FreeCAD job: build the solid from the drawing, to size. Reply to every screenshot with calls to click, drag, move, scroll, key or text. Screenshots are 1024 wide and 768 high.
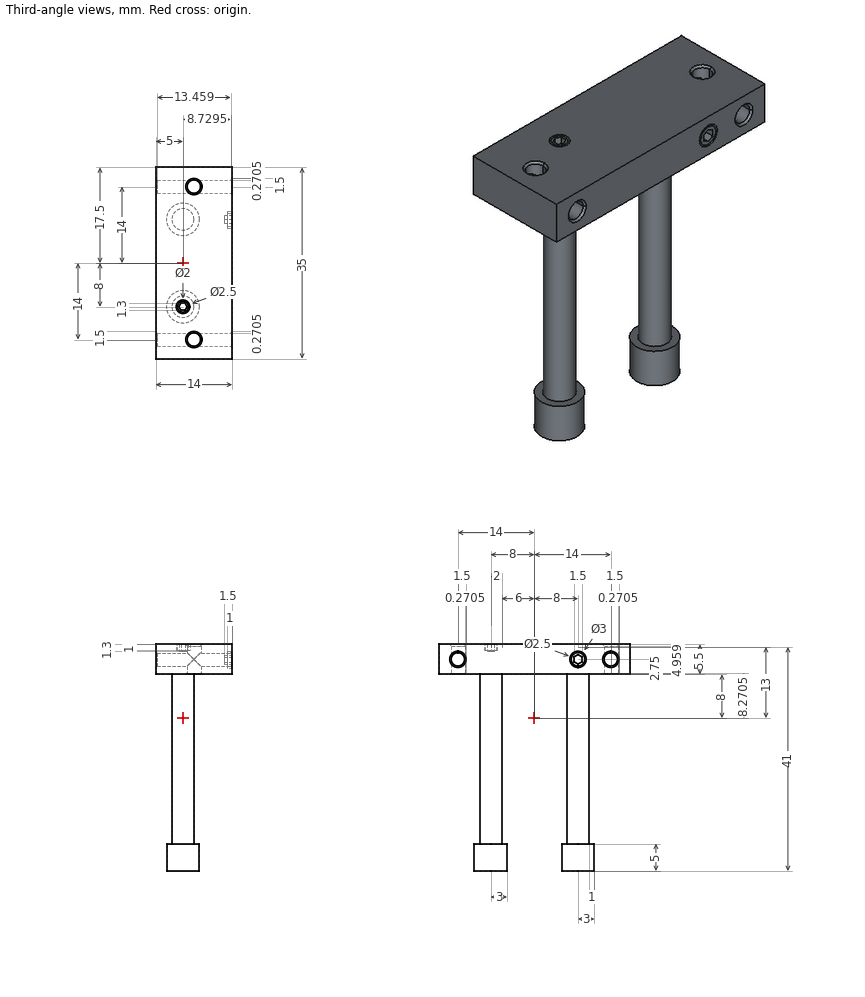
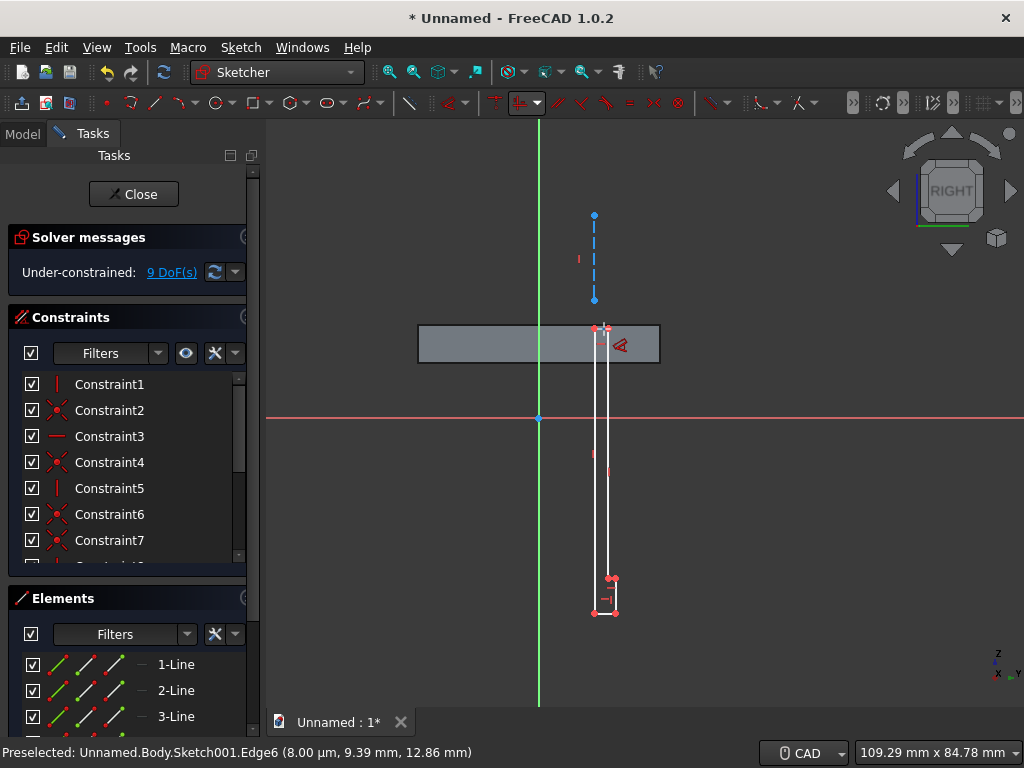
scroll(601, 614, up, 4)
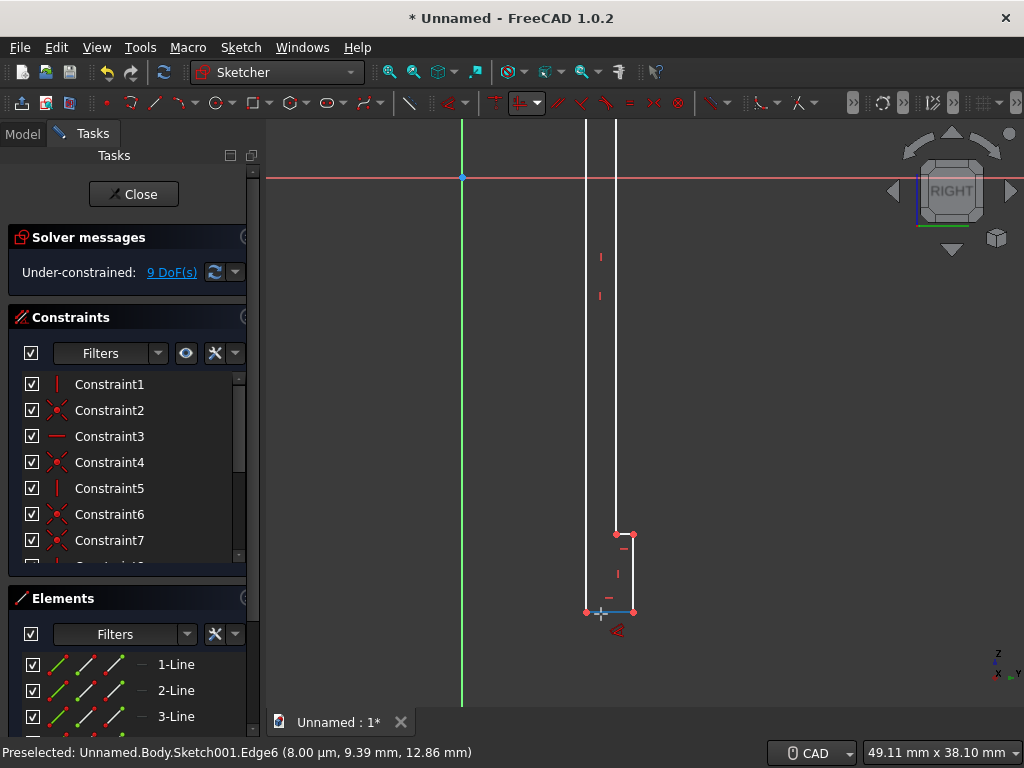
click(600, 612)
click(610, 646)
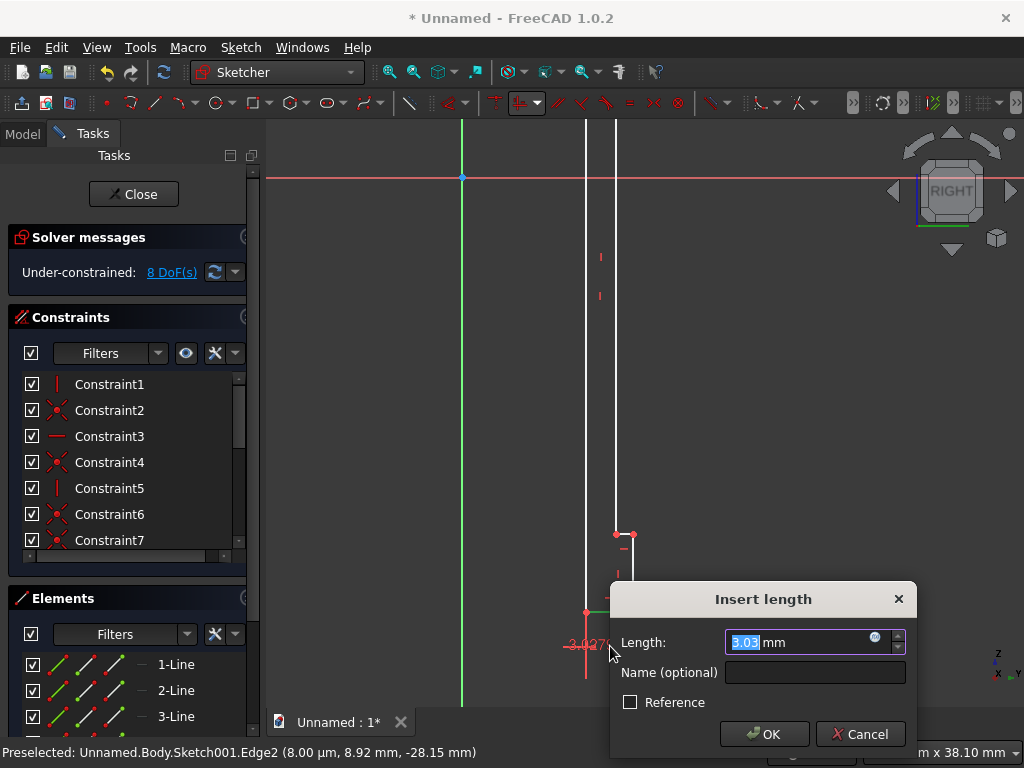
text(3)
key(Return)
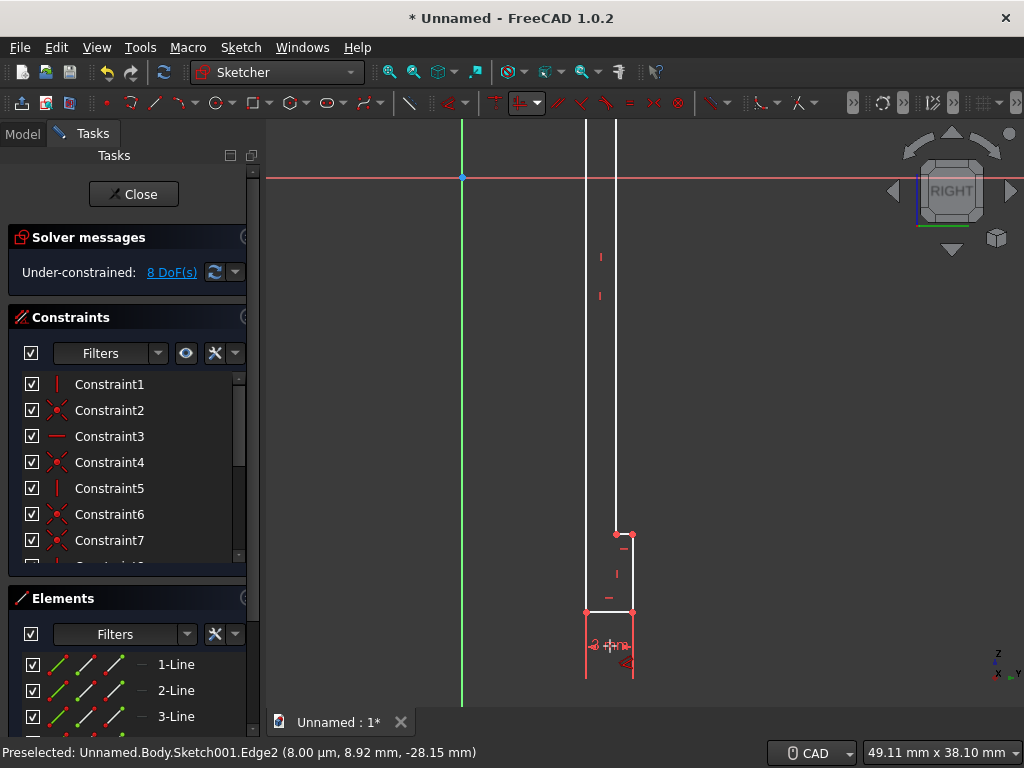
click(633, 589)
click(667, 573)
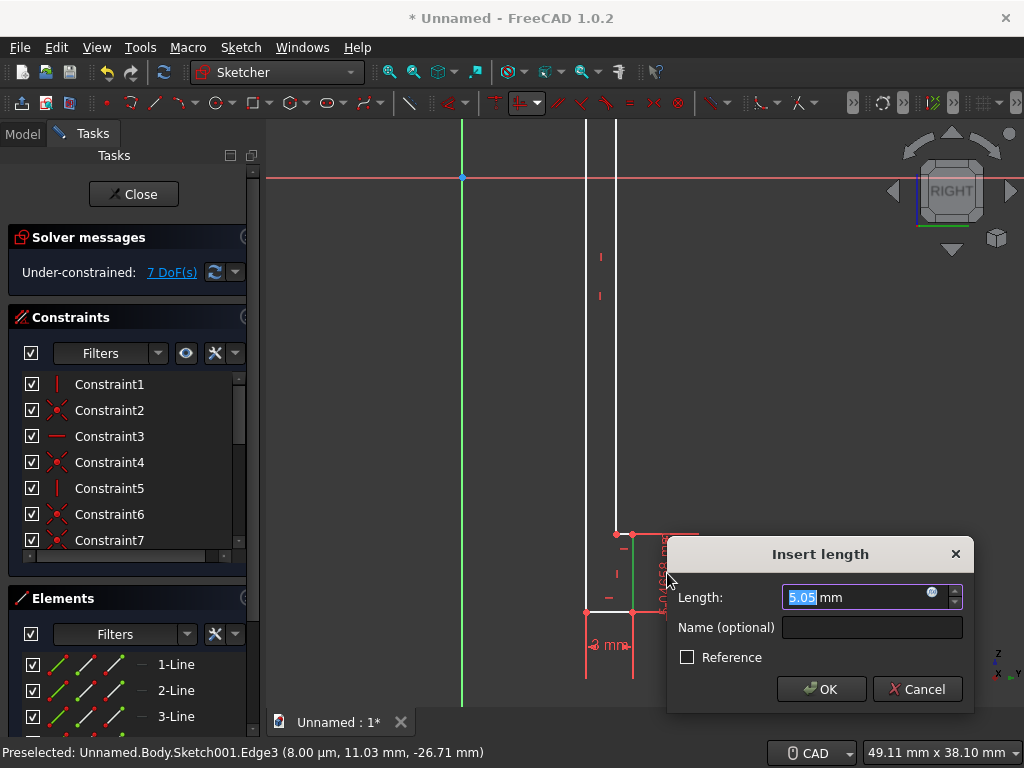
text(5)
key(Return)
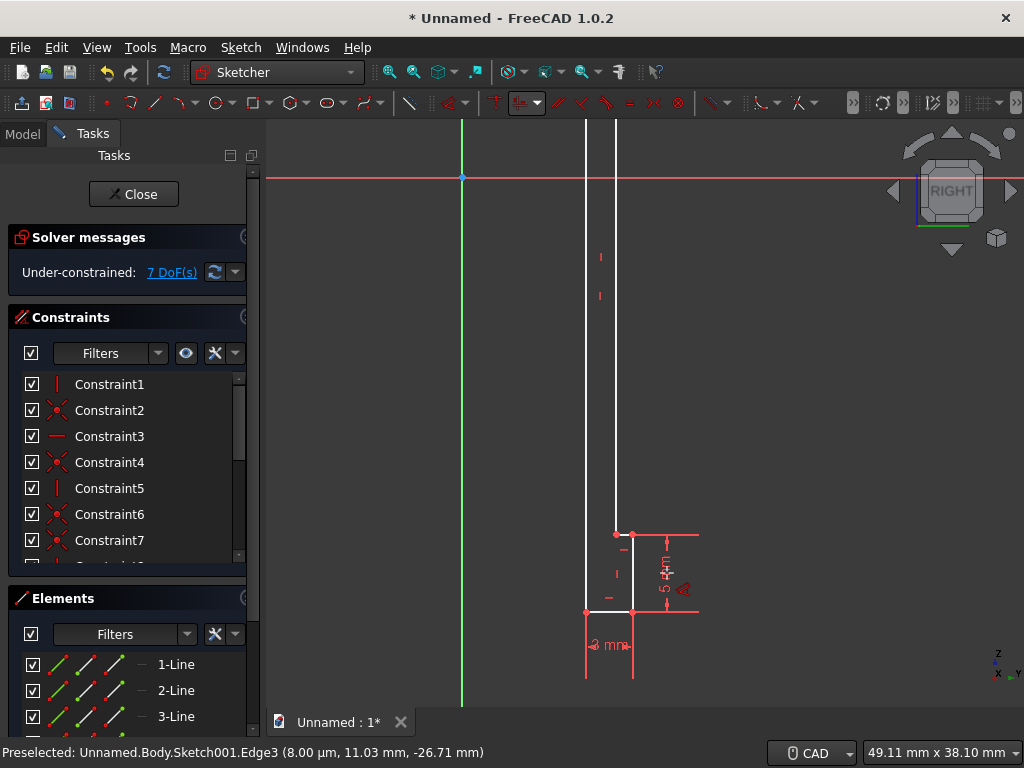
scroll(625, 535, up, 5)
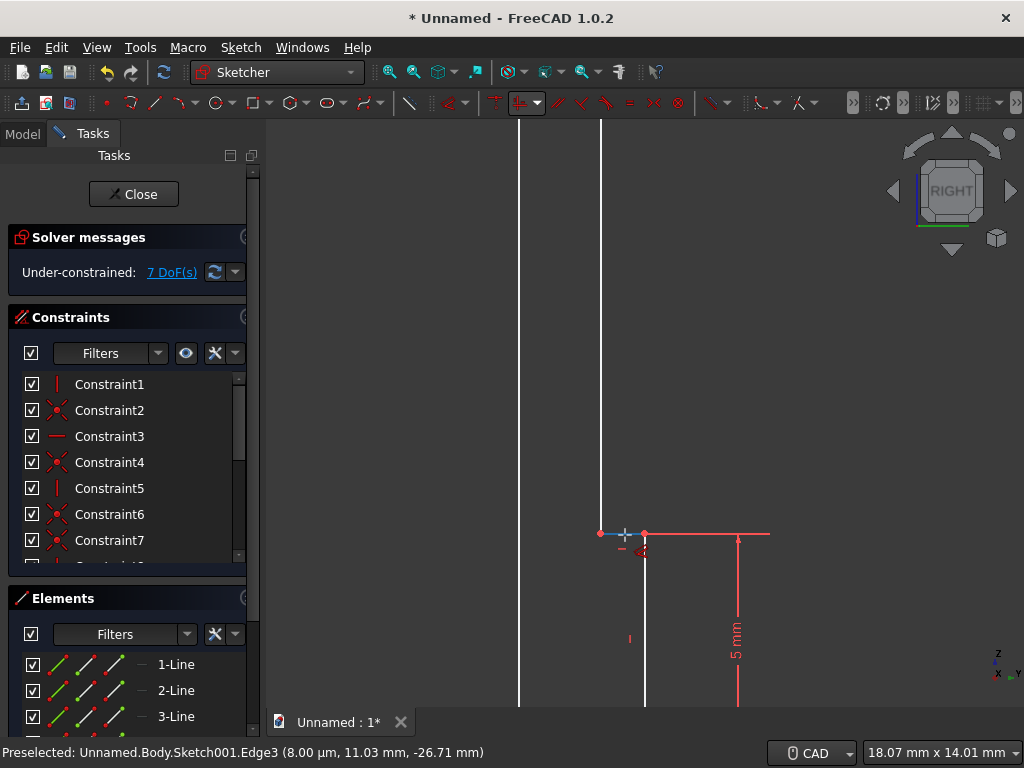
click(623, 534)
click(623, 568)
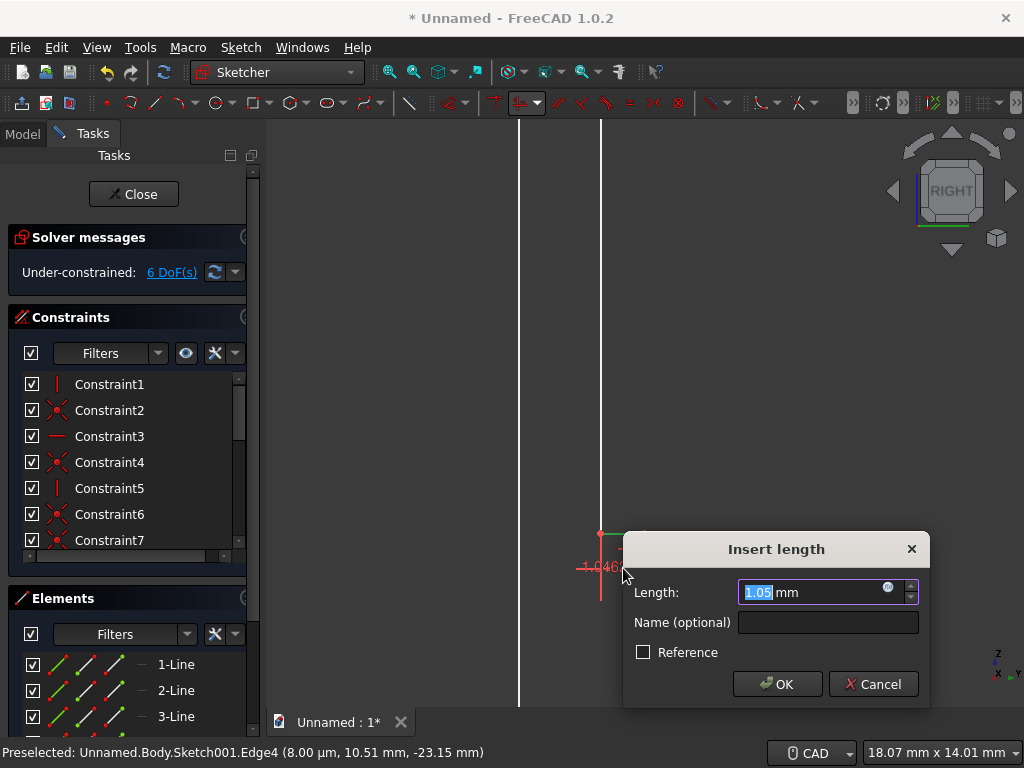
text(1)
key(Return)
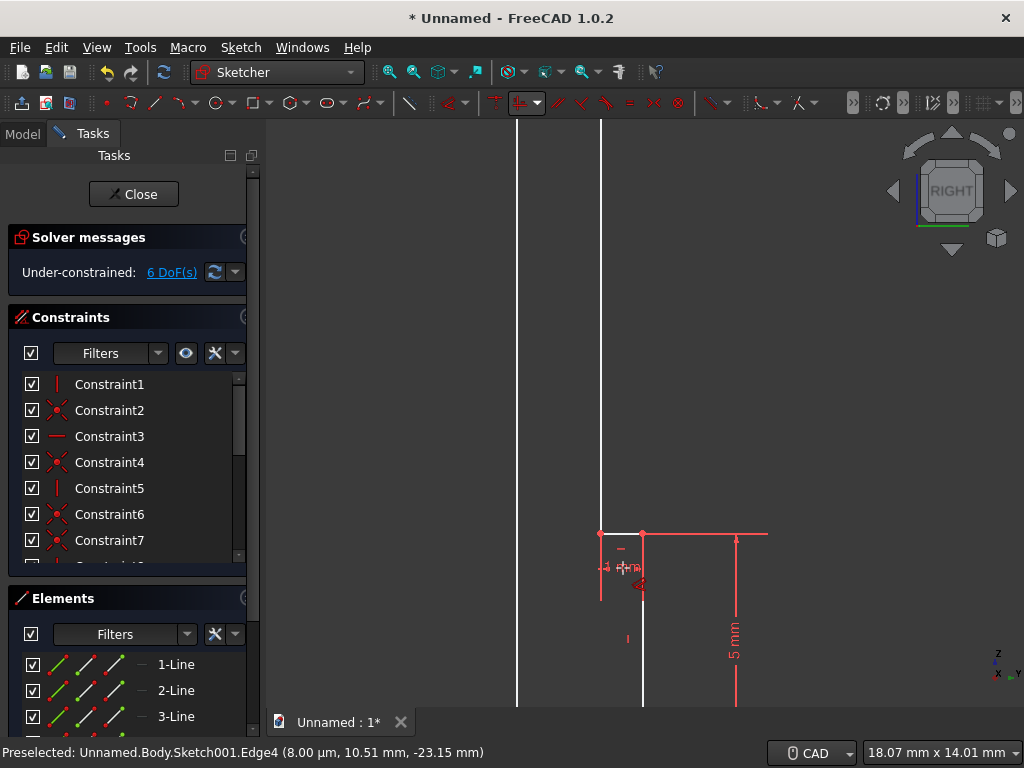
scroll(609, 587, down, 9)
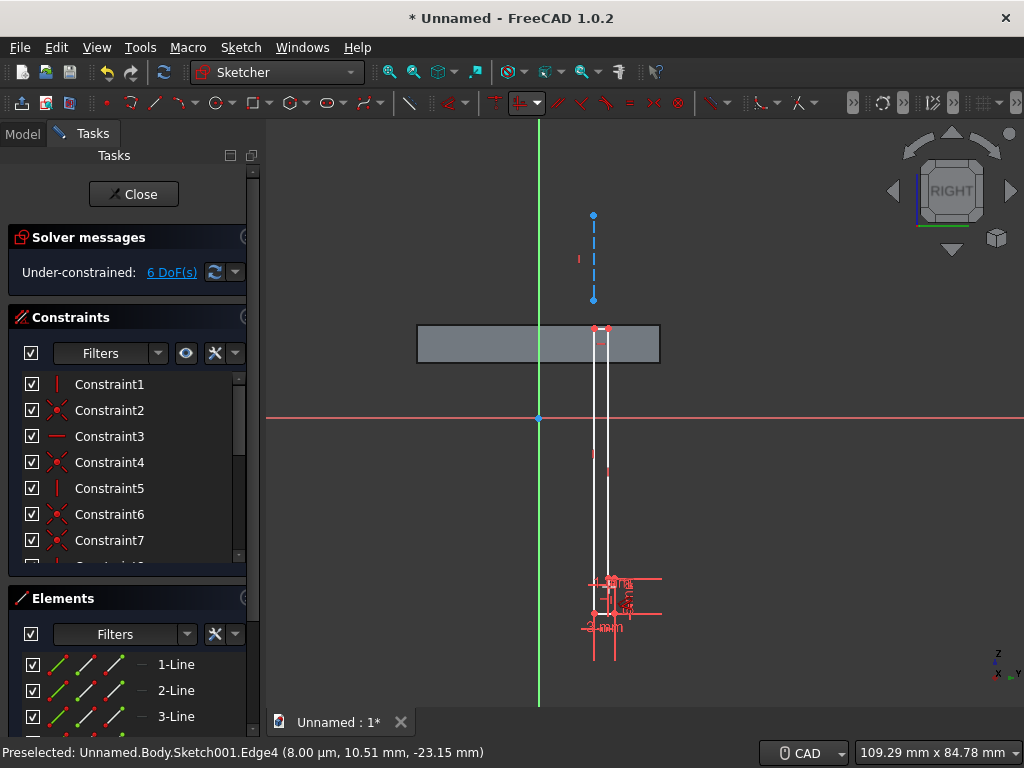
click(594, 528)
click(628, 471)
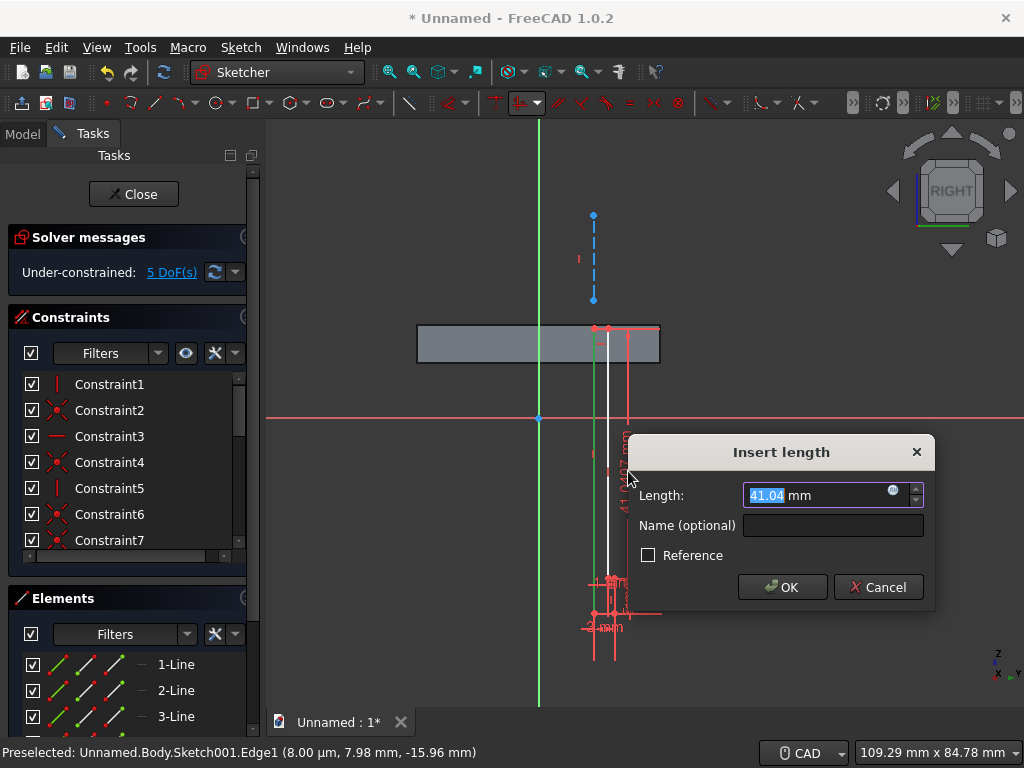
text(41)
key(Return)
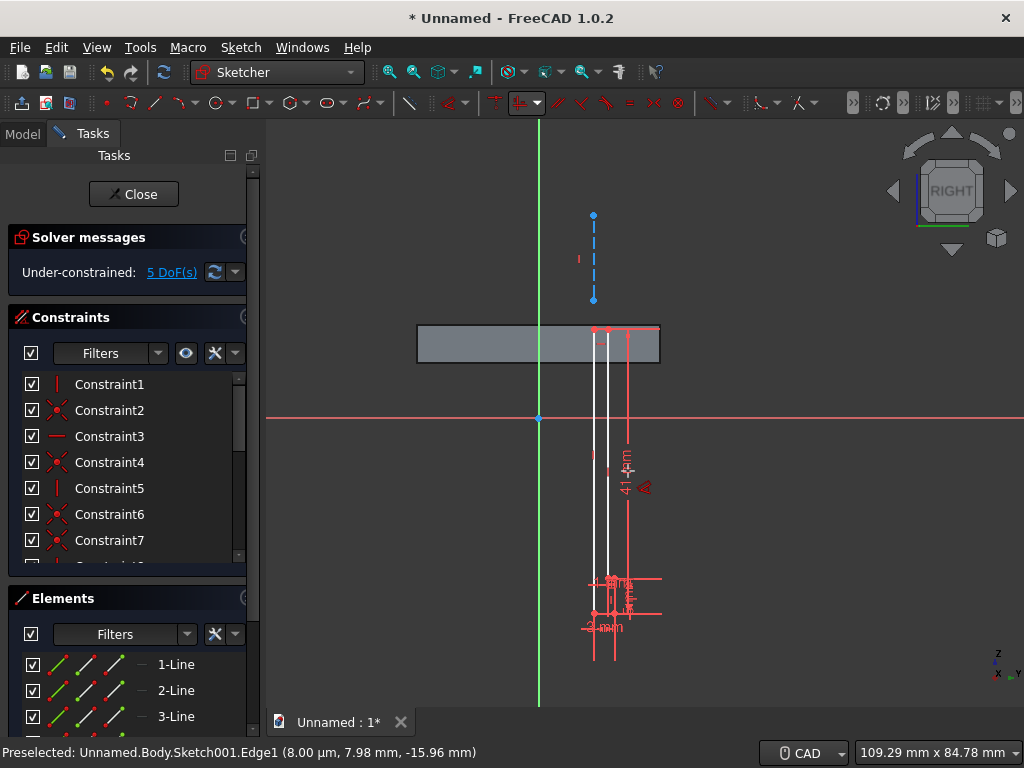
click(594, 329)
click(566, 295)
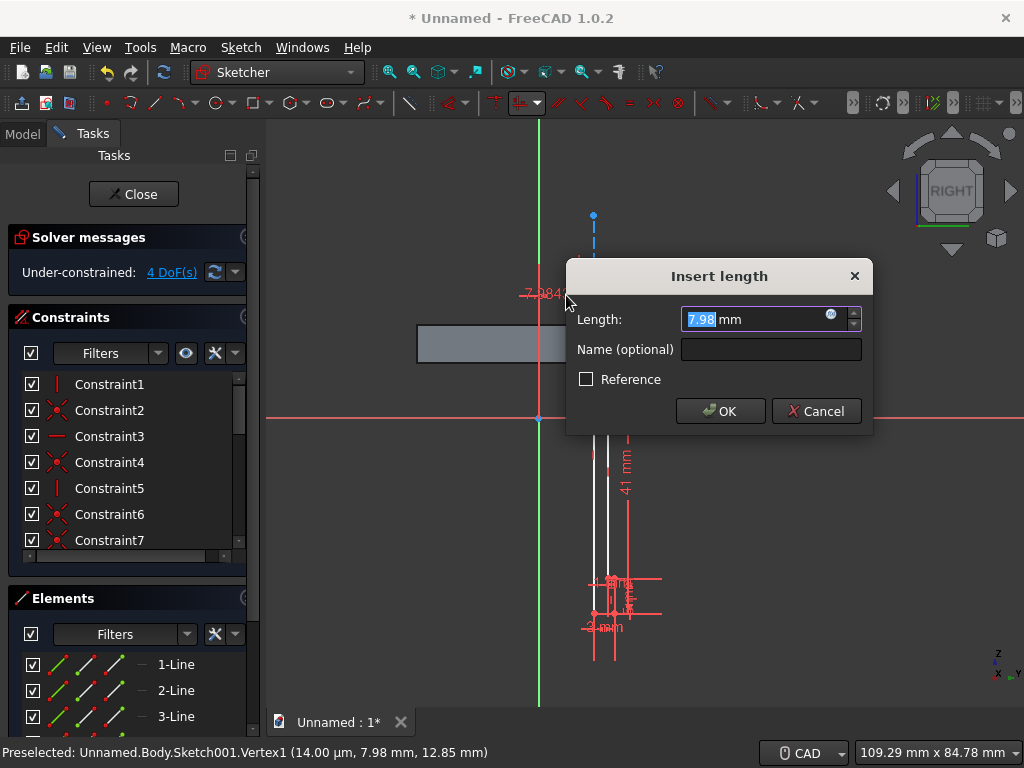
text(8)
key(Return)